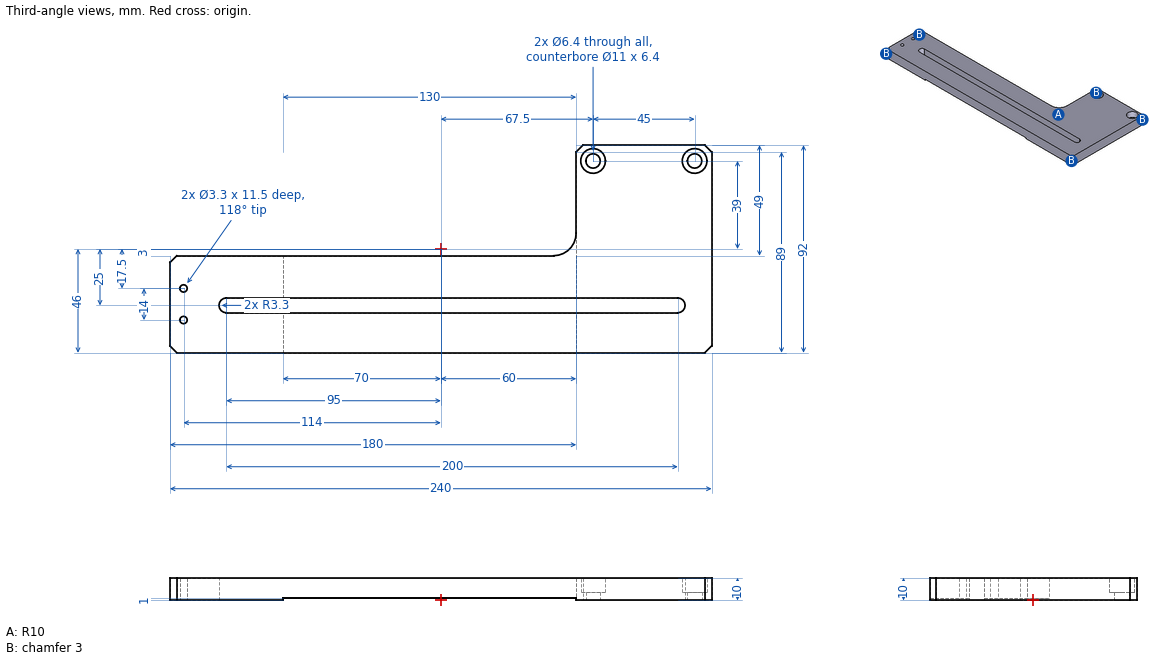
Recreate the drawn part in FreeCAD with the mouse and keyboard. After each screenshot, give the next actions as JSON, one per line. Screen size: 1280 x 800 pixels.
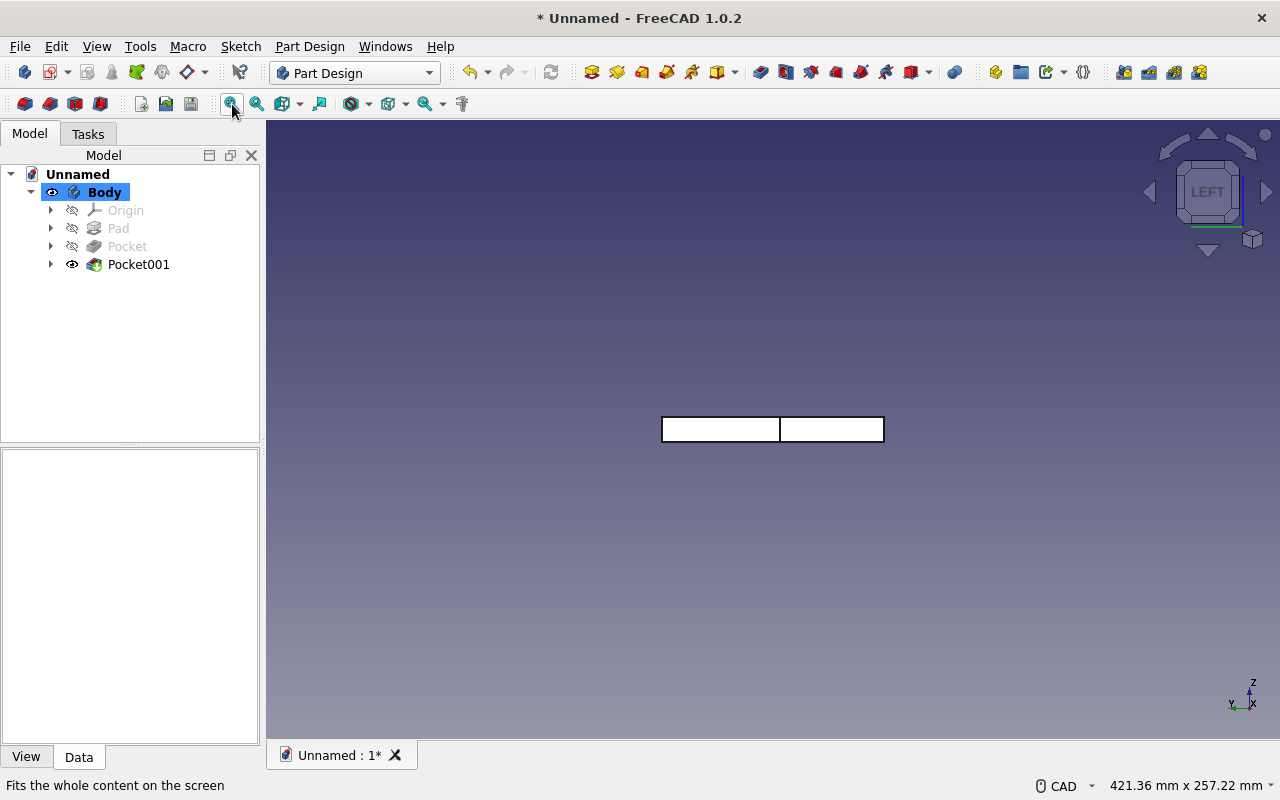
{"action": "key", "text": "v 3"}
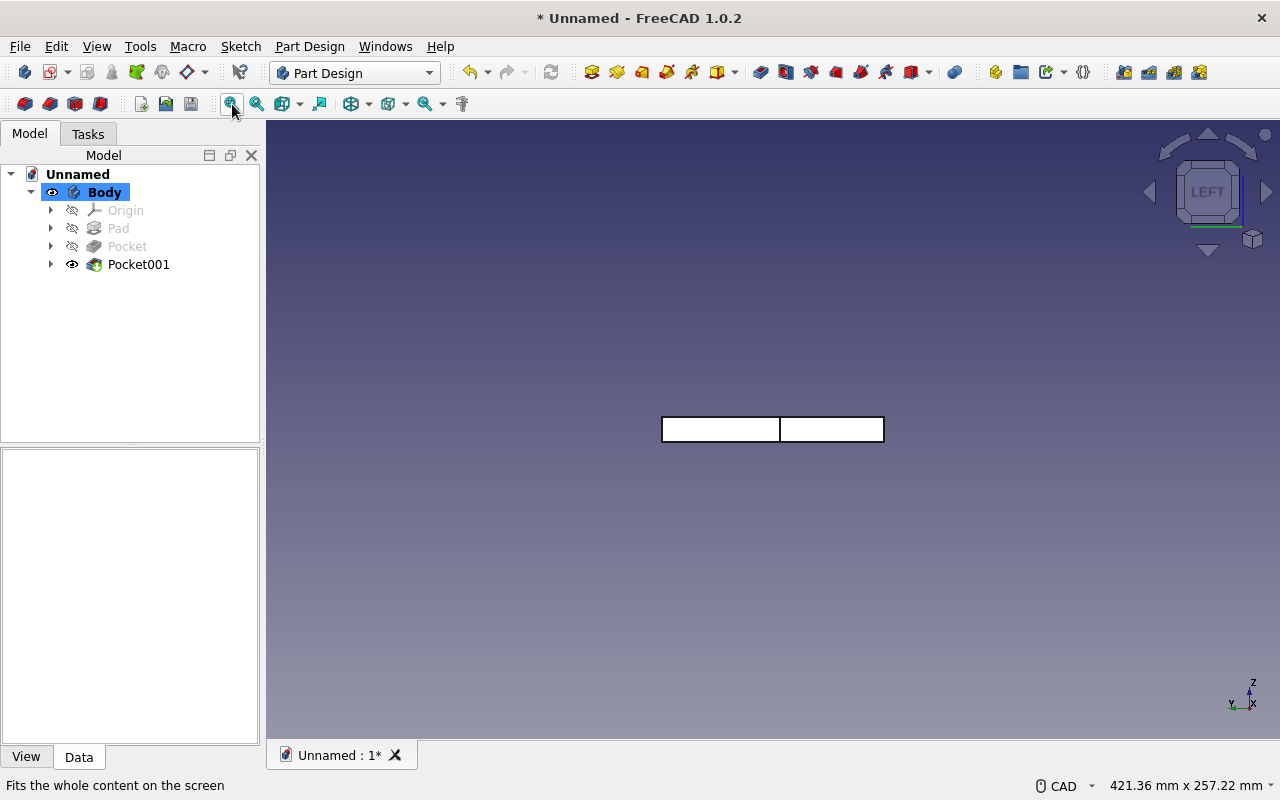
{"action": "key", "text": "0"}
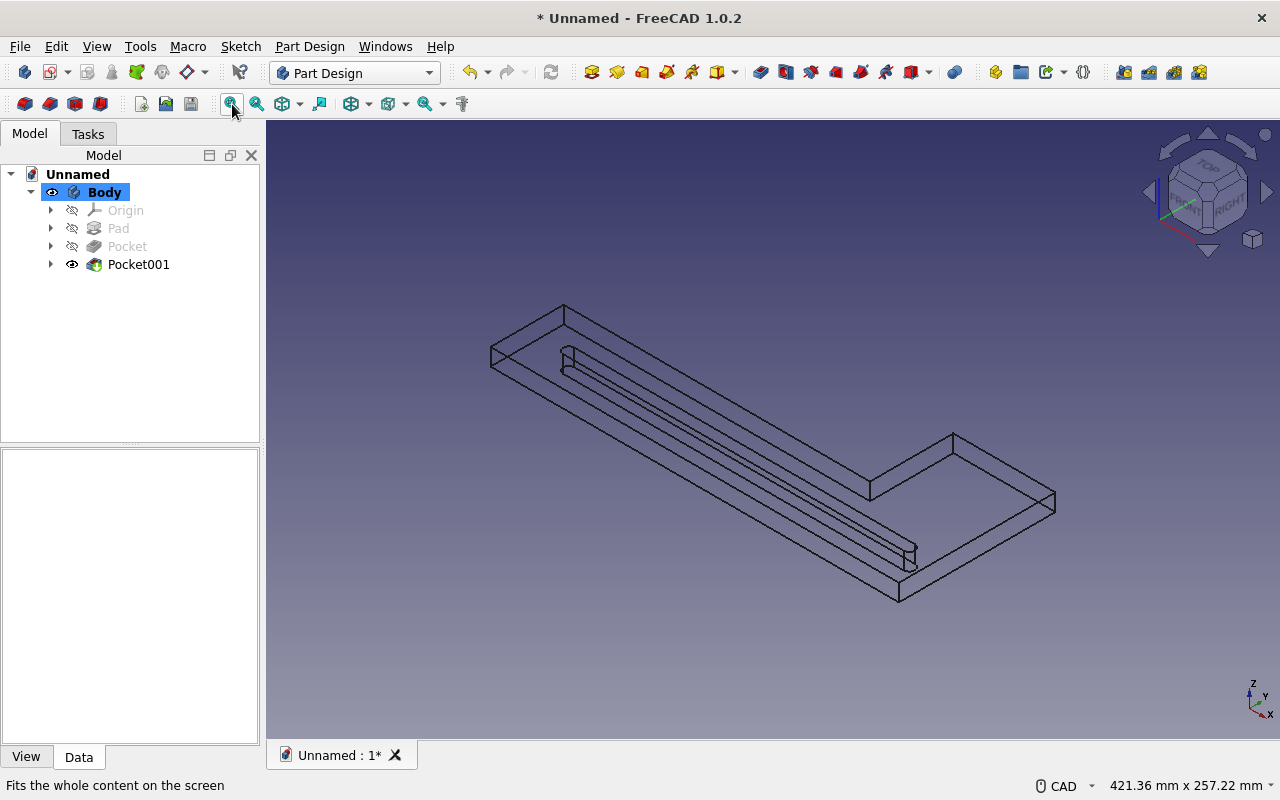
{"action": "left_click", "coordinate": [870, 490]}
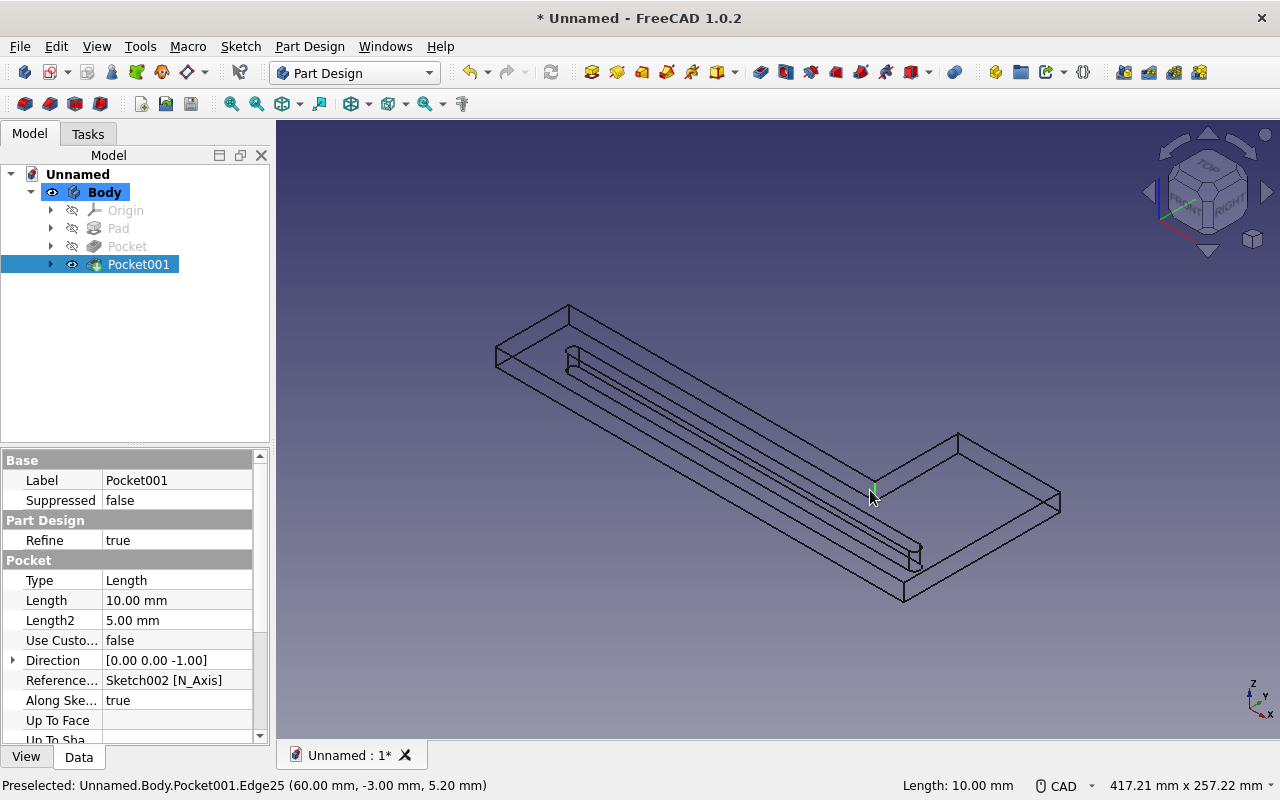
{"action": "key", "text": "v 1"}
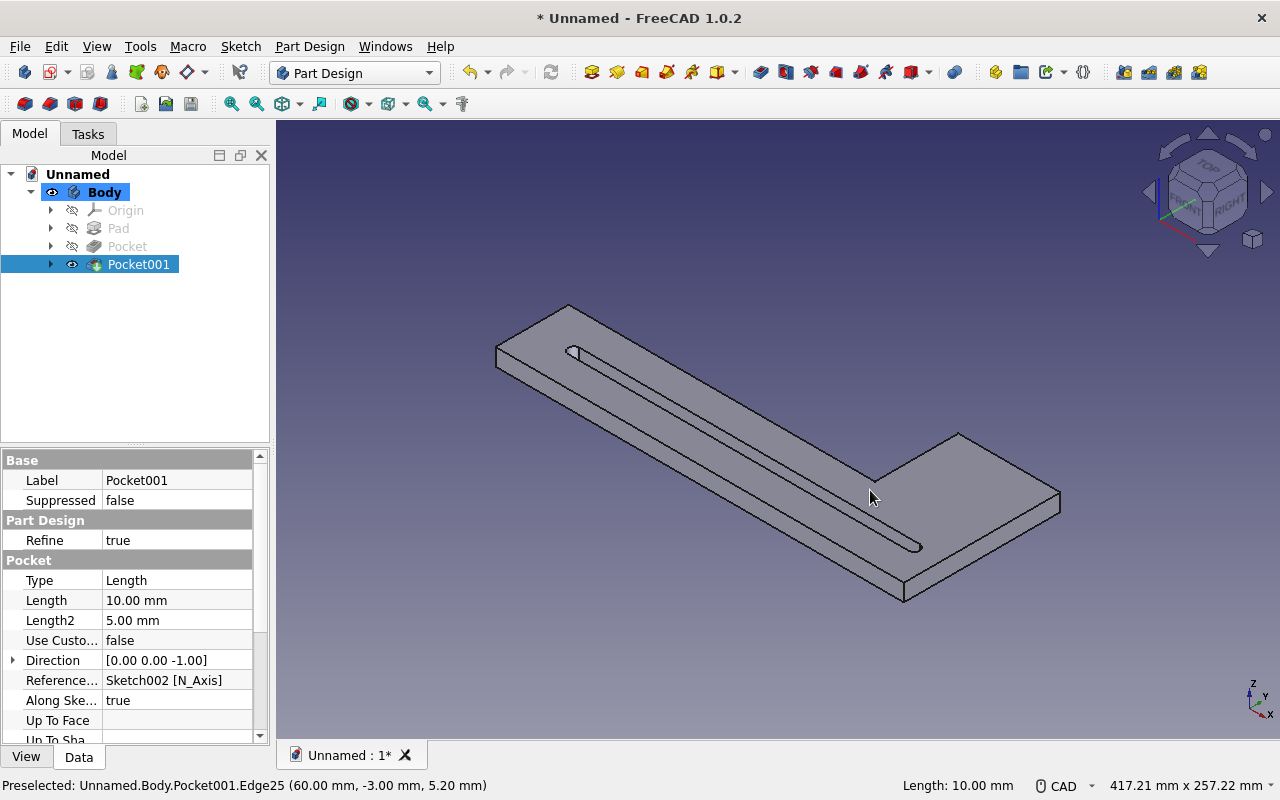
{"action": "left_click", "coordinate": [25, 104]}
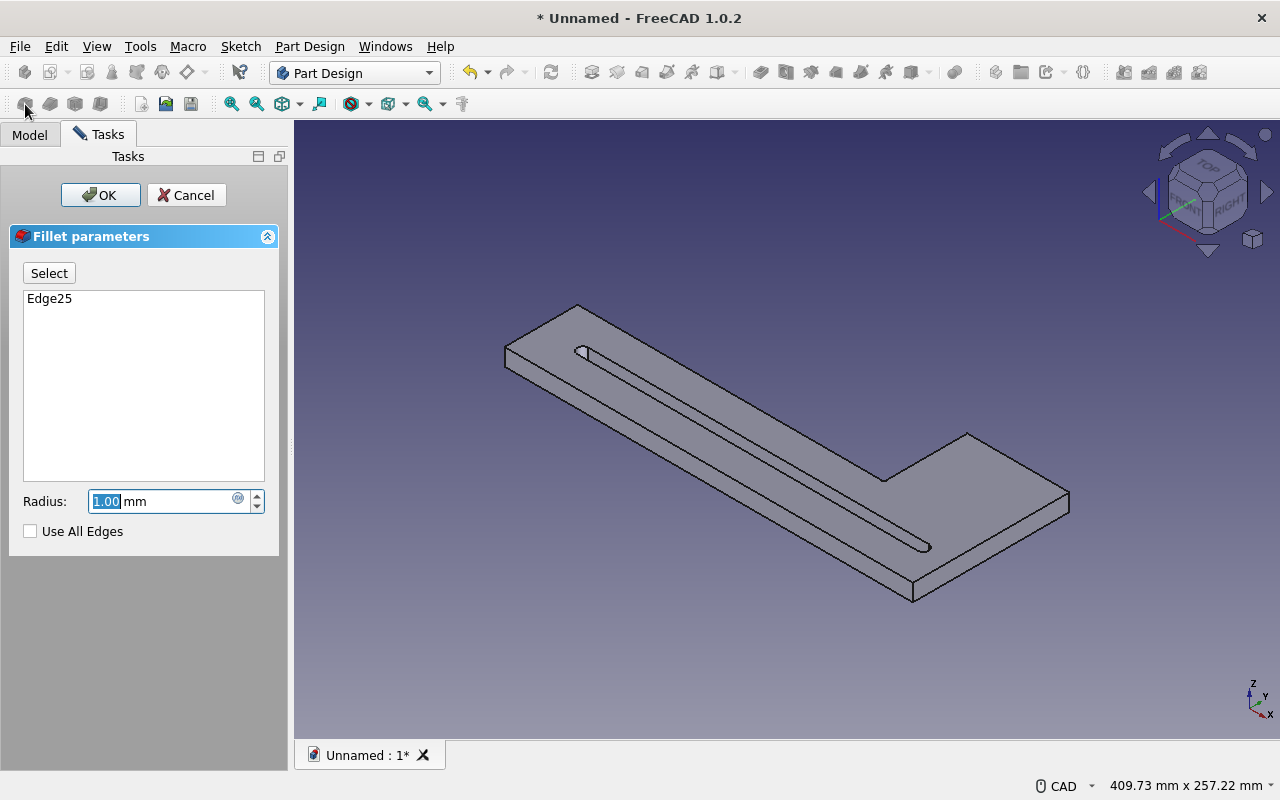
{"action": "type", "text": "10"}
{"action": "key", "text": "Tab"}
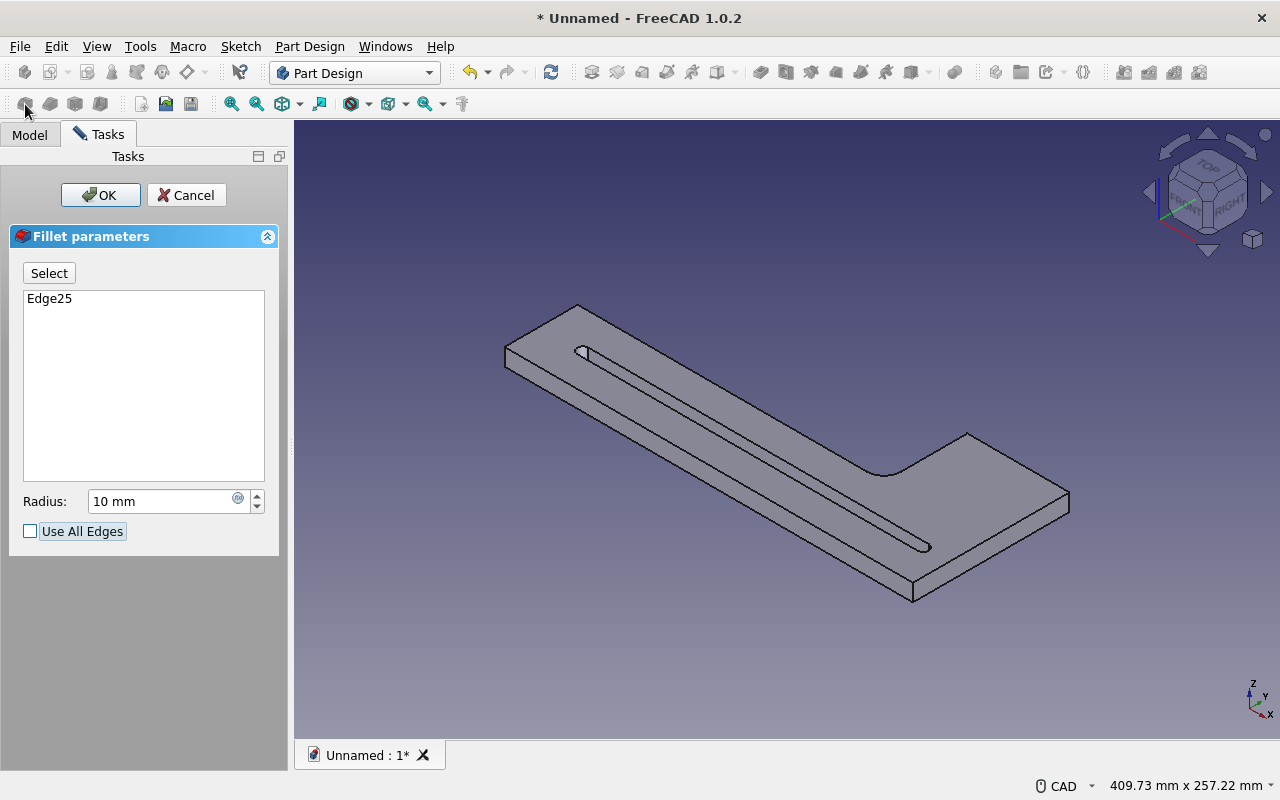
{"action": "left_click", "coordinate": [101, 195]}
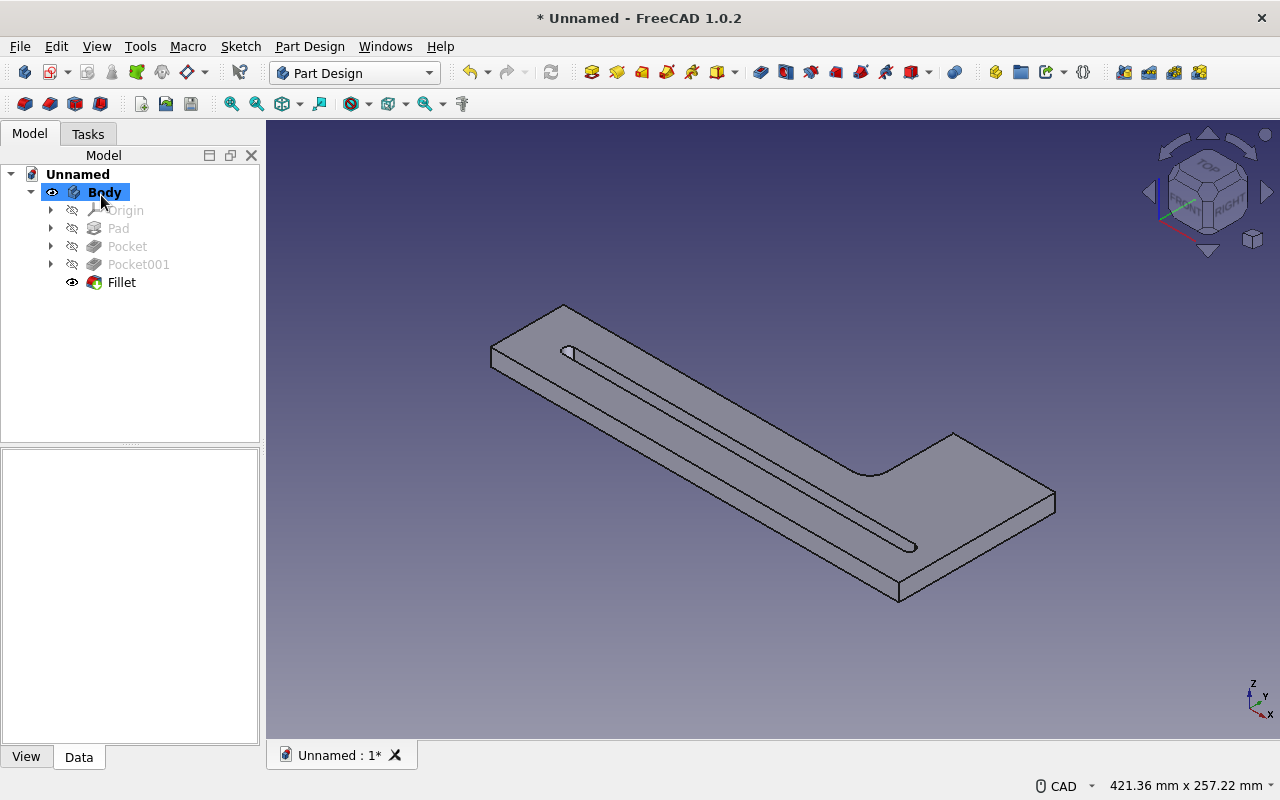
{"action": "left_click", "coordinate": [899, 592]}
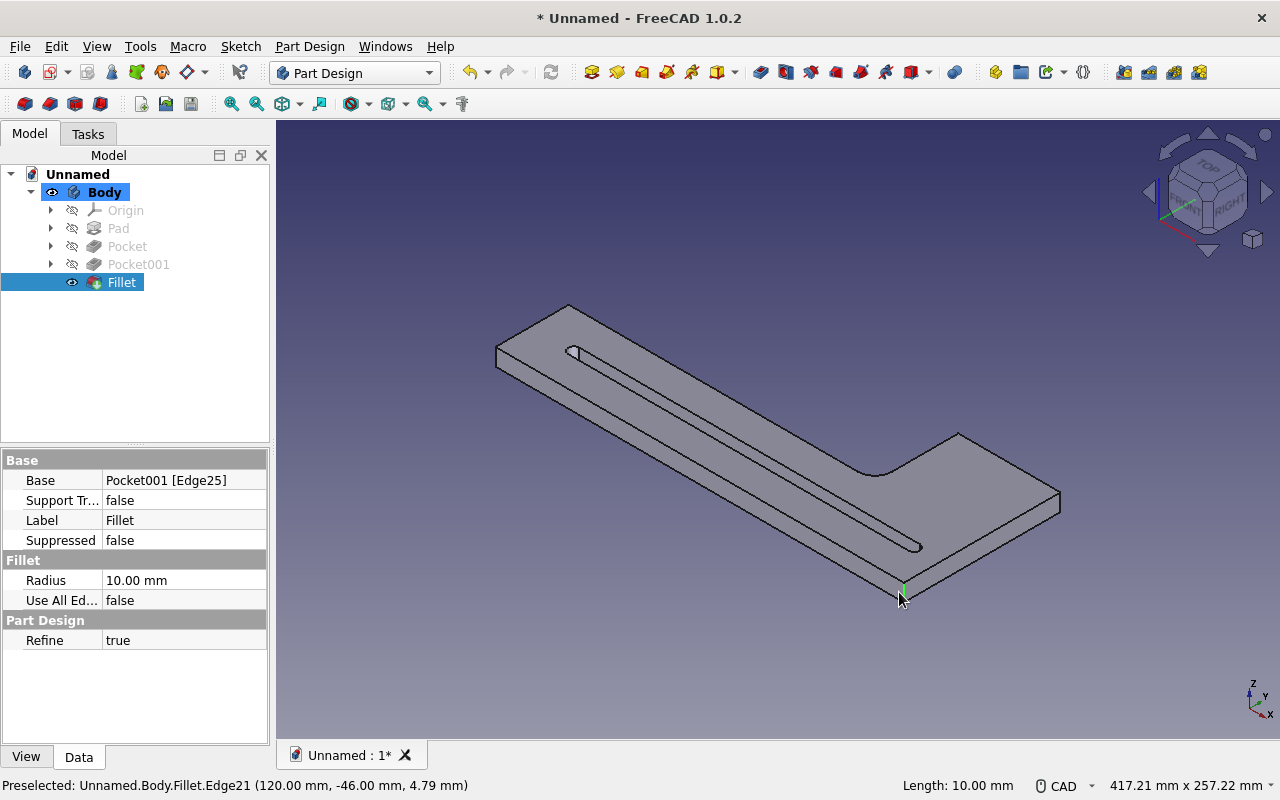
{"action": "key", "text": "2"}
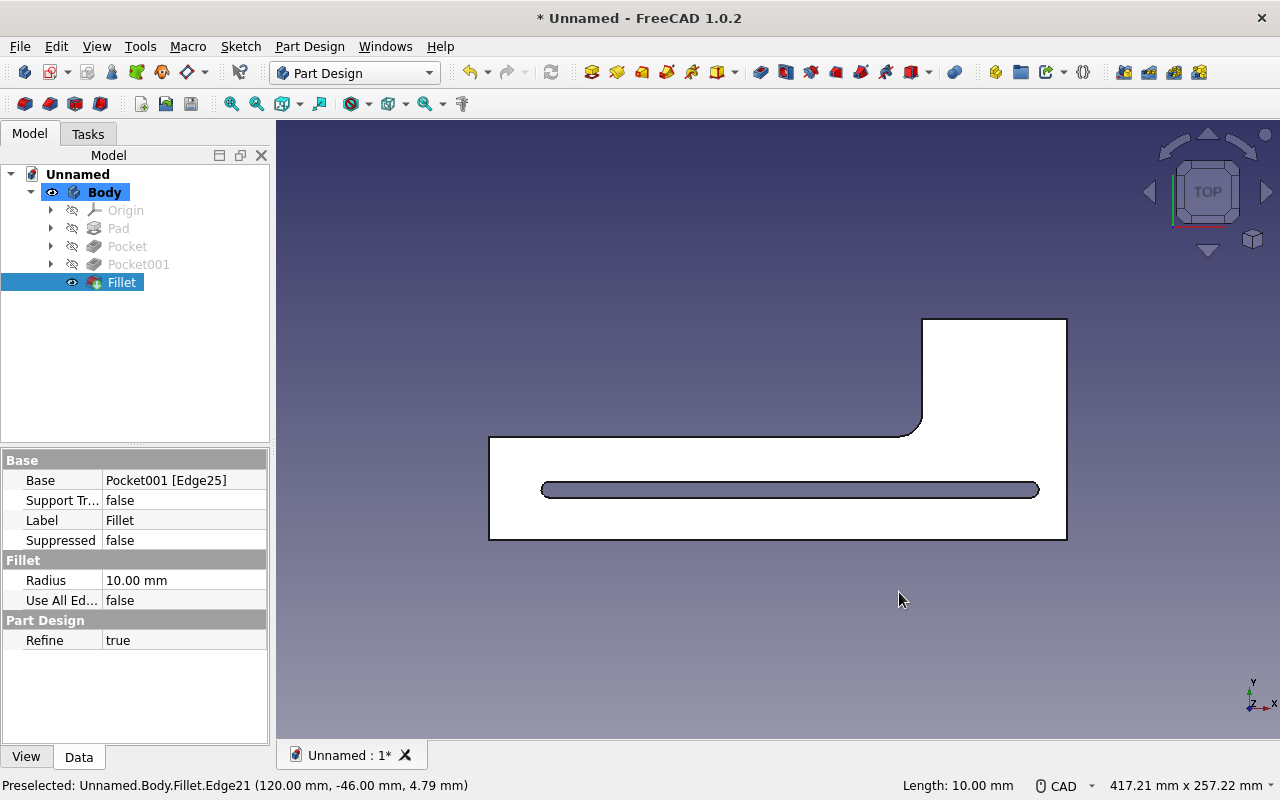
{"action": "key", "text": "0"}